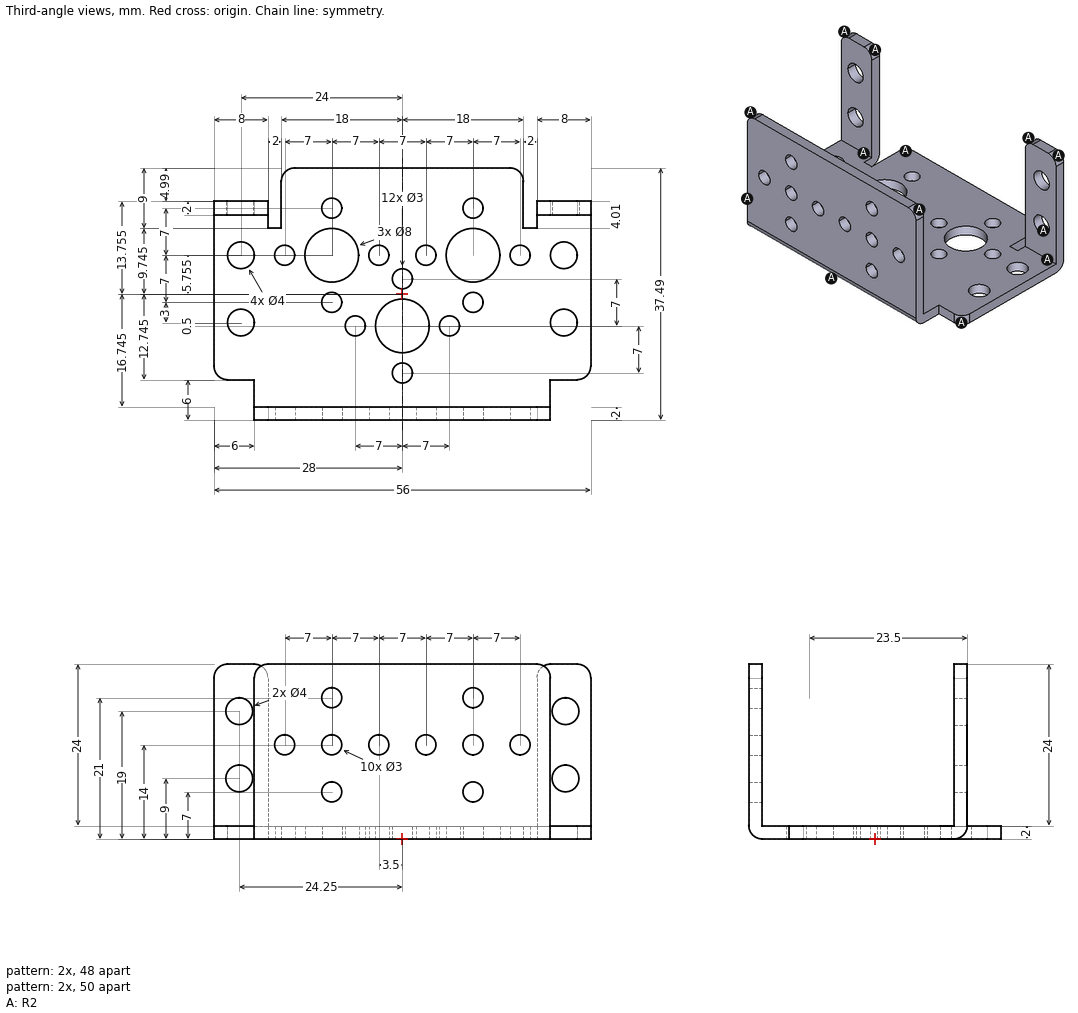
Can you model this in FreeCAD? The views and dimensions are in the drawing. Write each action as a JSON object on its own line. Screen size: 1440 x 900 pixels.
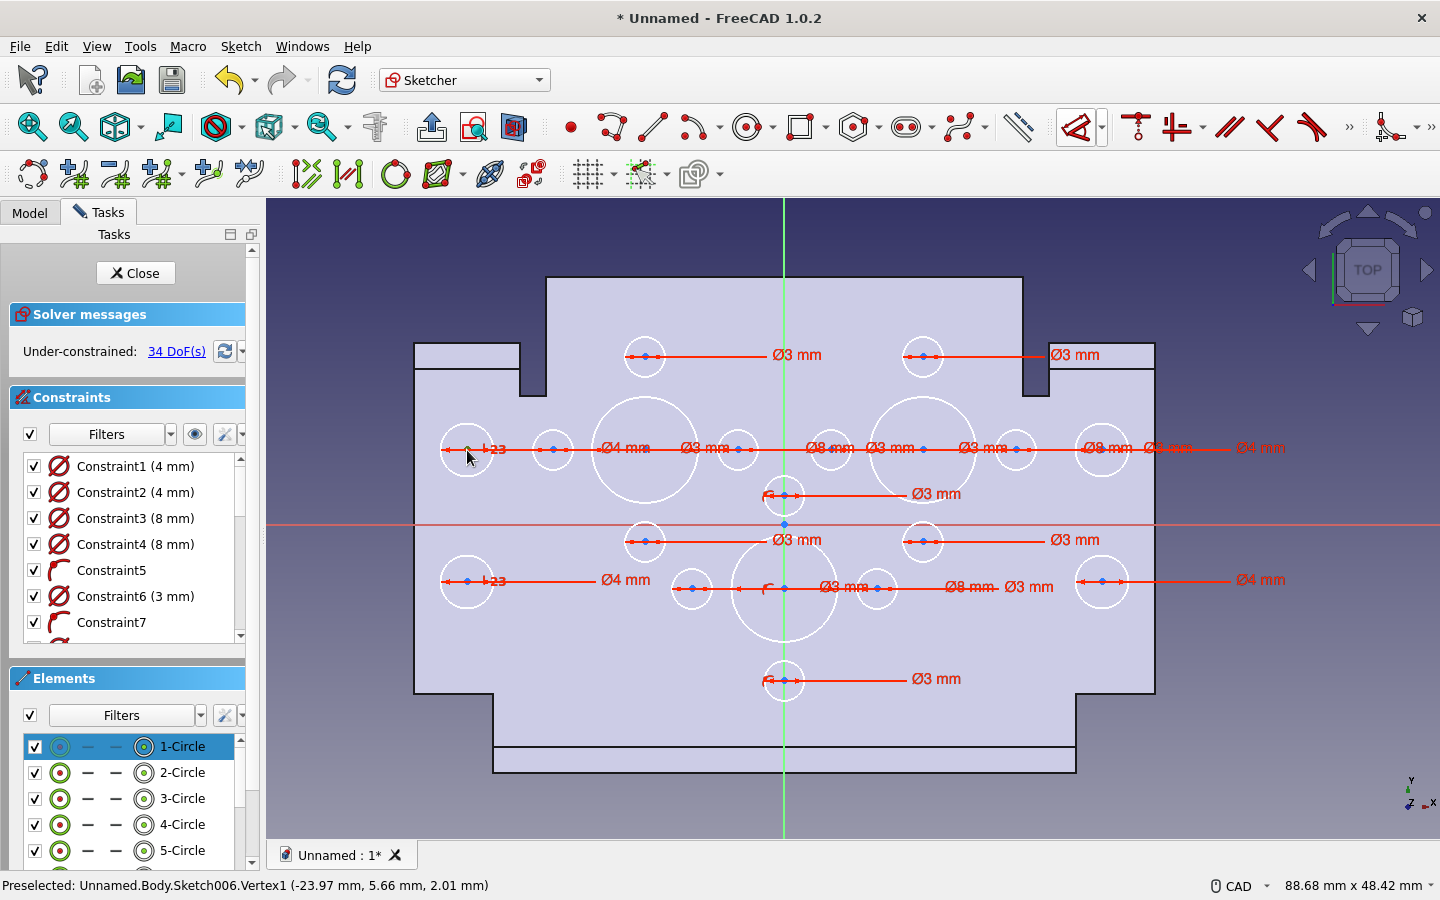
{"action": "left_click", "coordinate": [645, 450]}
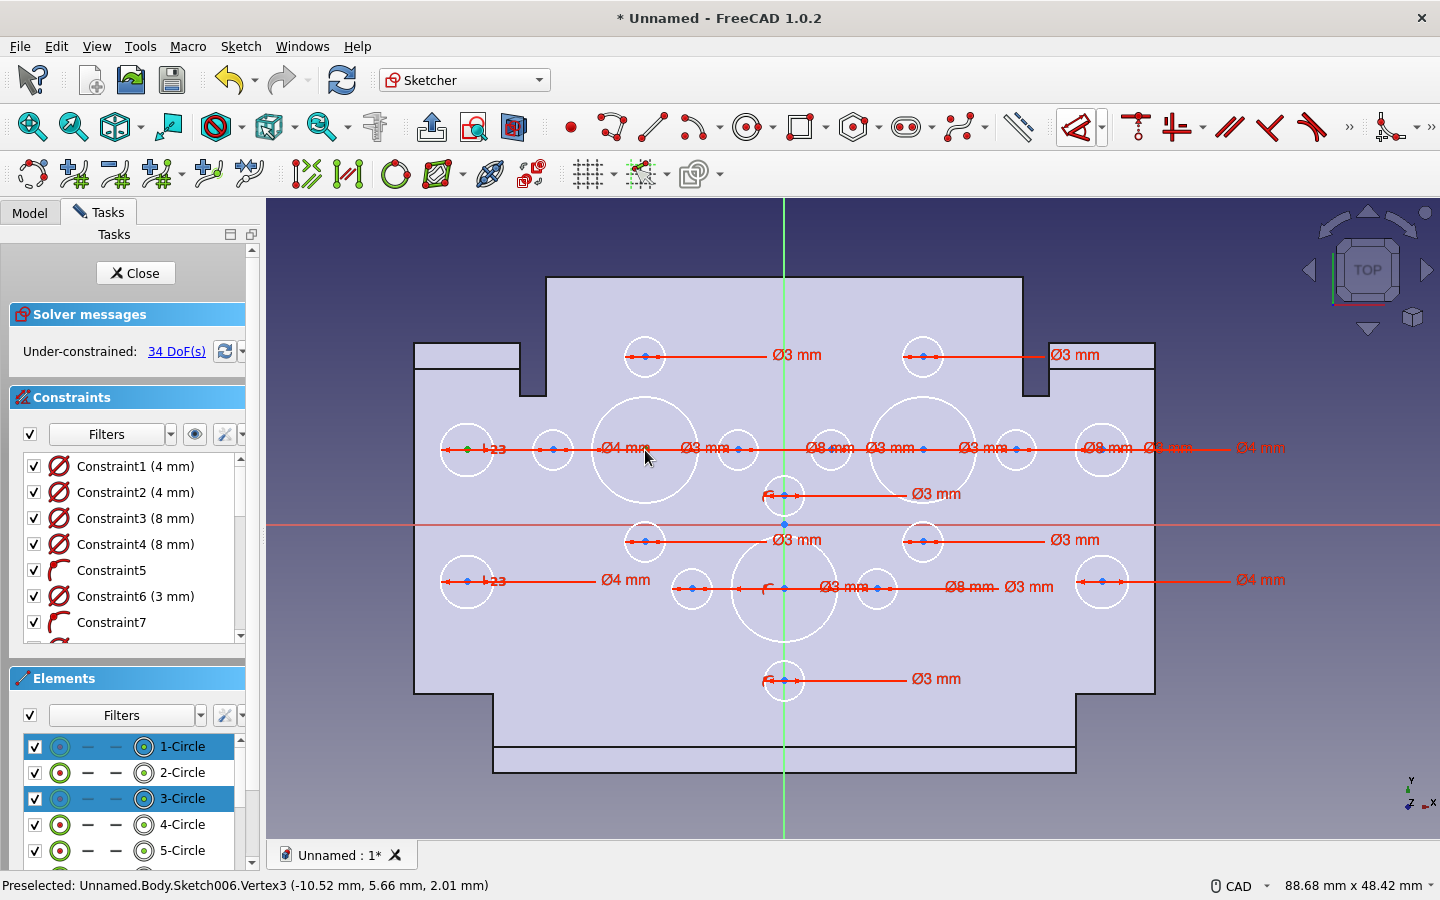
{"action": "key", "text": "h"}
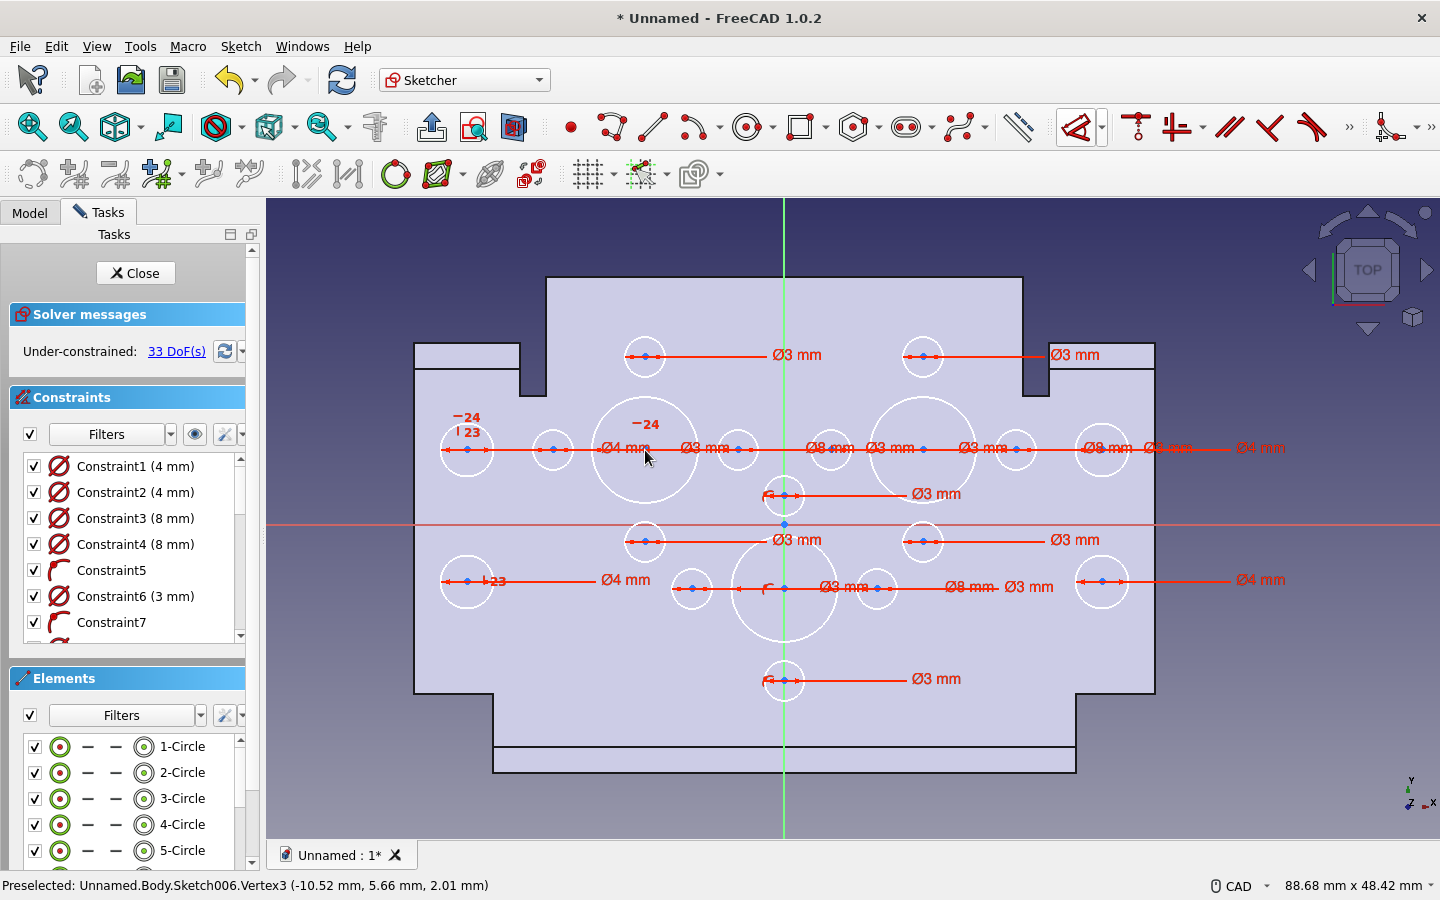
{"action": "left_click", "coordinate": [645, 450]}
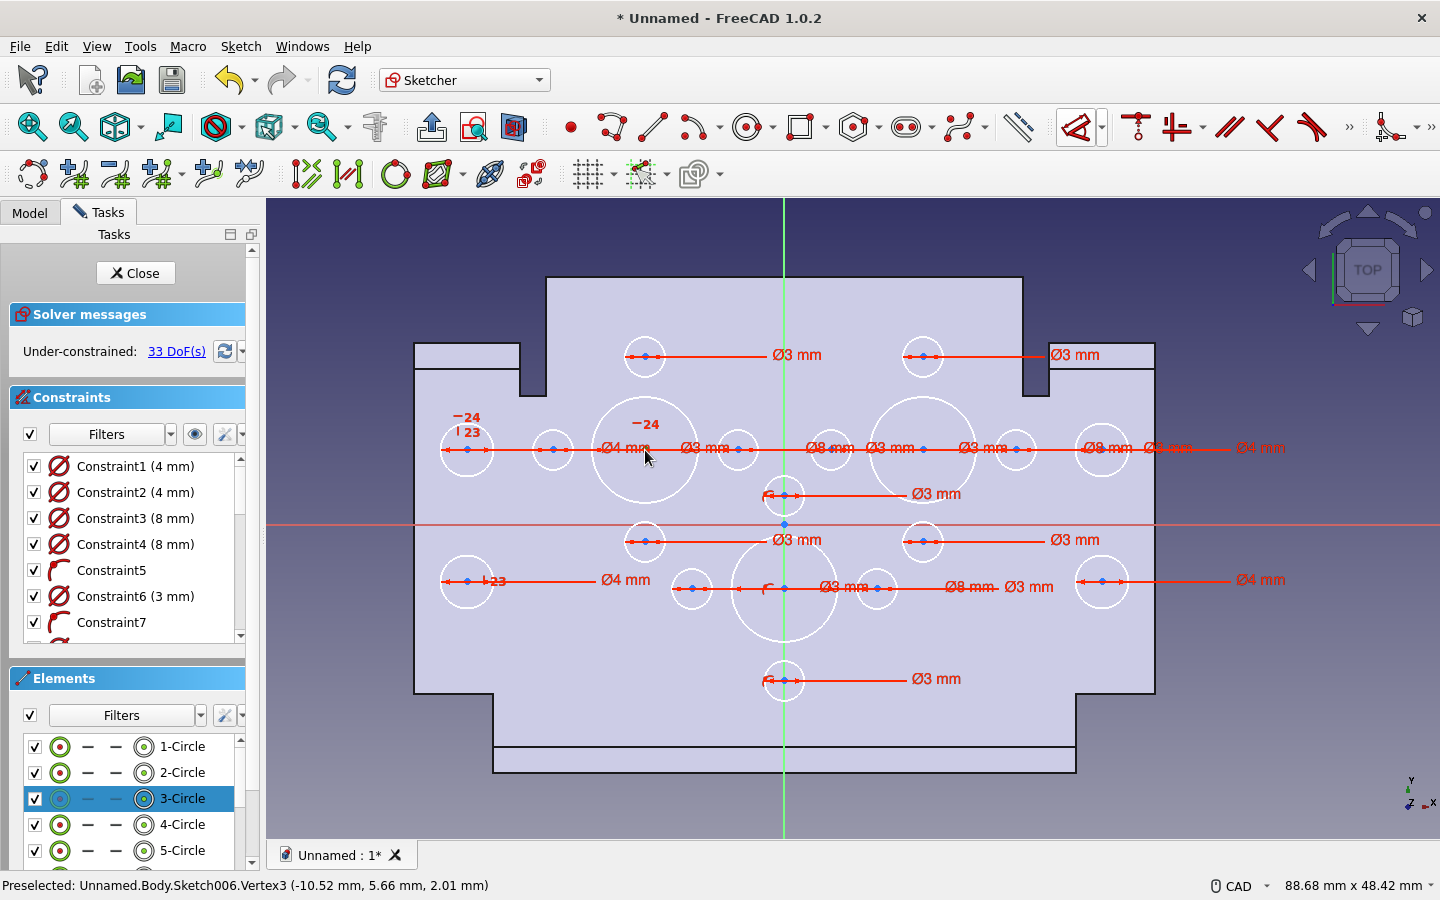
{"action": "left_click", "coordinate": [645, 542]}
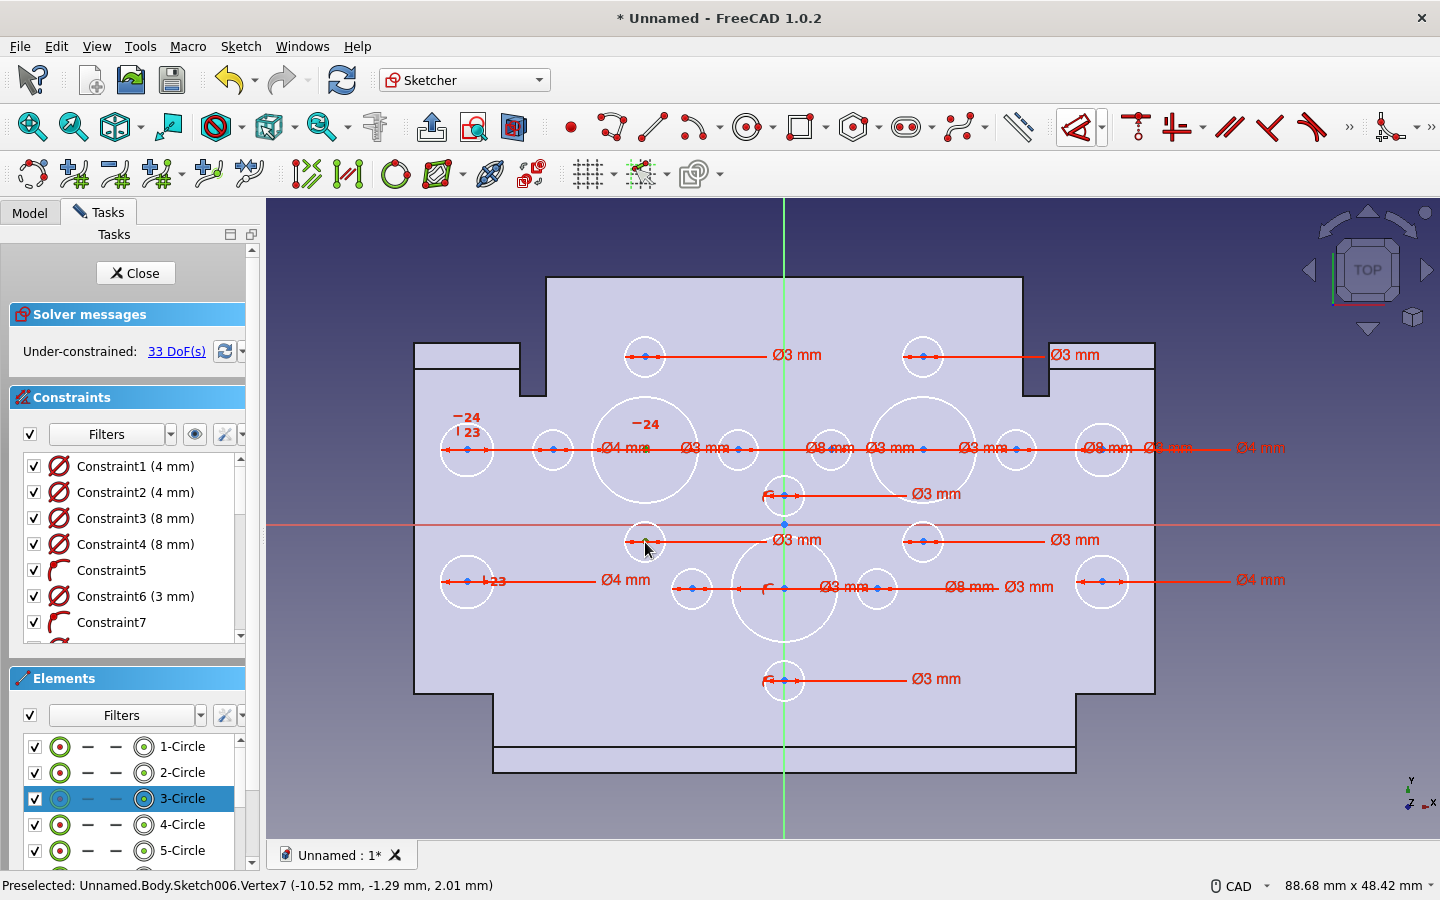
{"action": "key", "text": "v"}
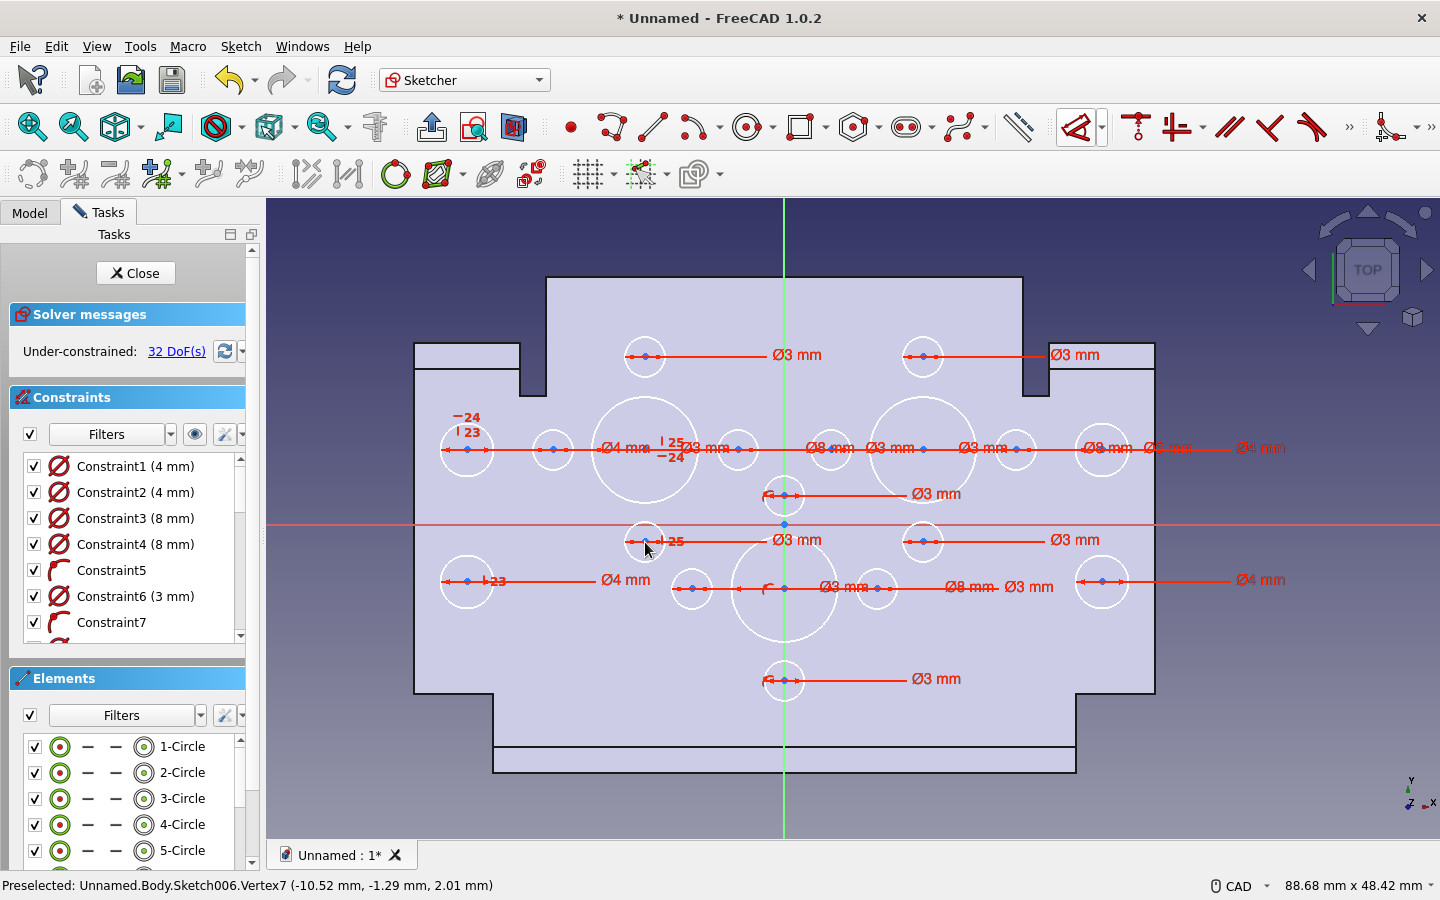
{"action": "left_click", "coordinate": [645, 450]}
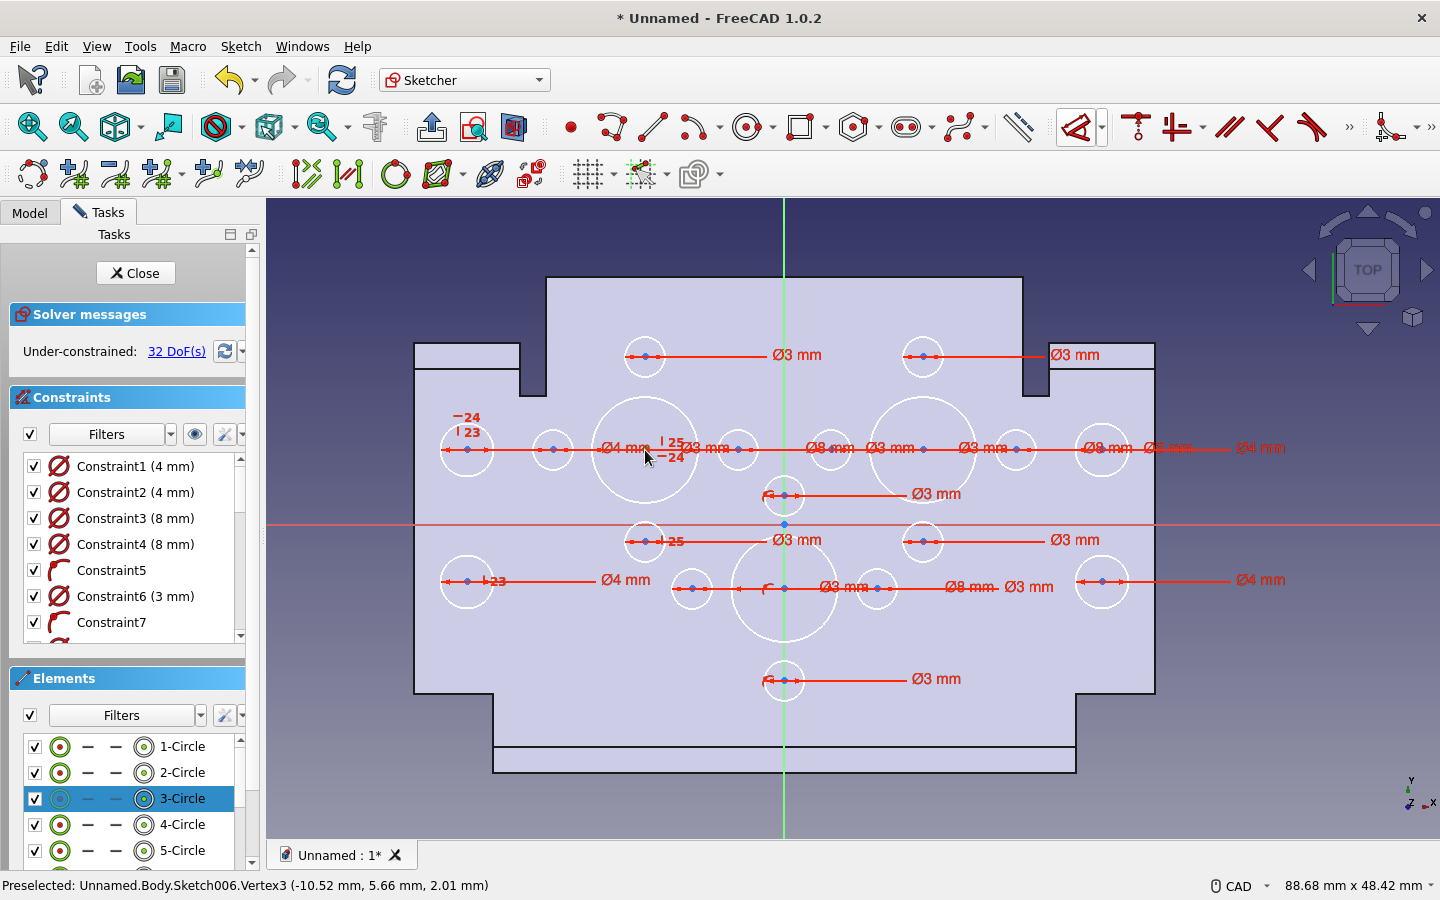
{"action": "left_click", "coordinate": [645, 357]}